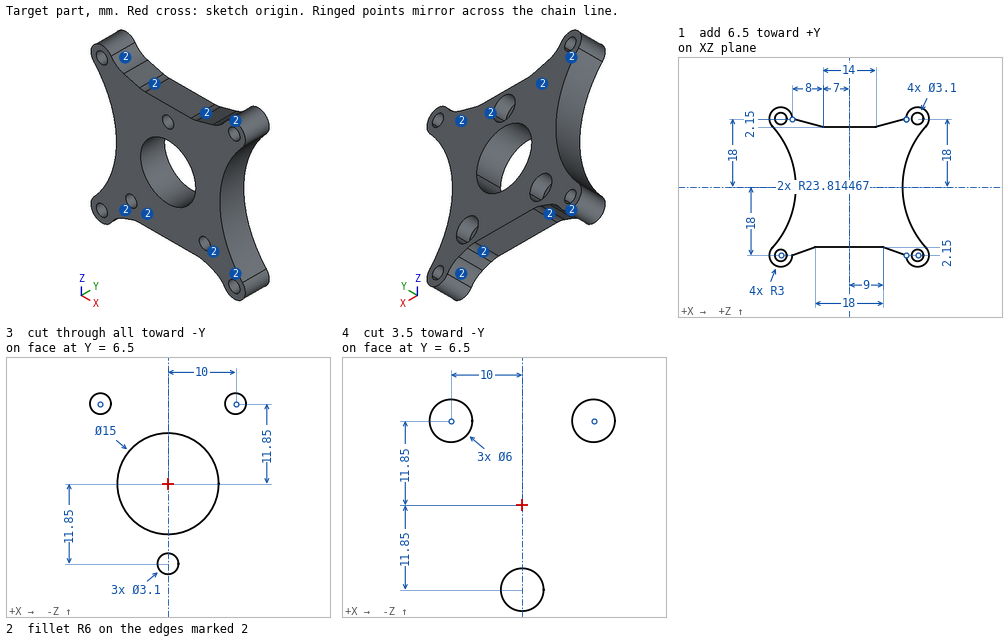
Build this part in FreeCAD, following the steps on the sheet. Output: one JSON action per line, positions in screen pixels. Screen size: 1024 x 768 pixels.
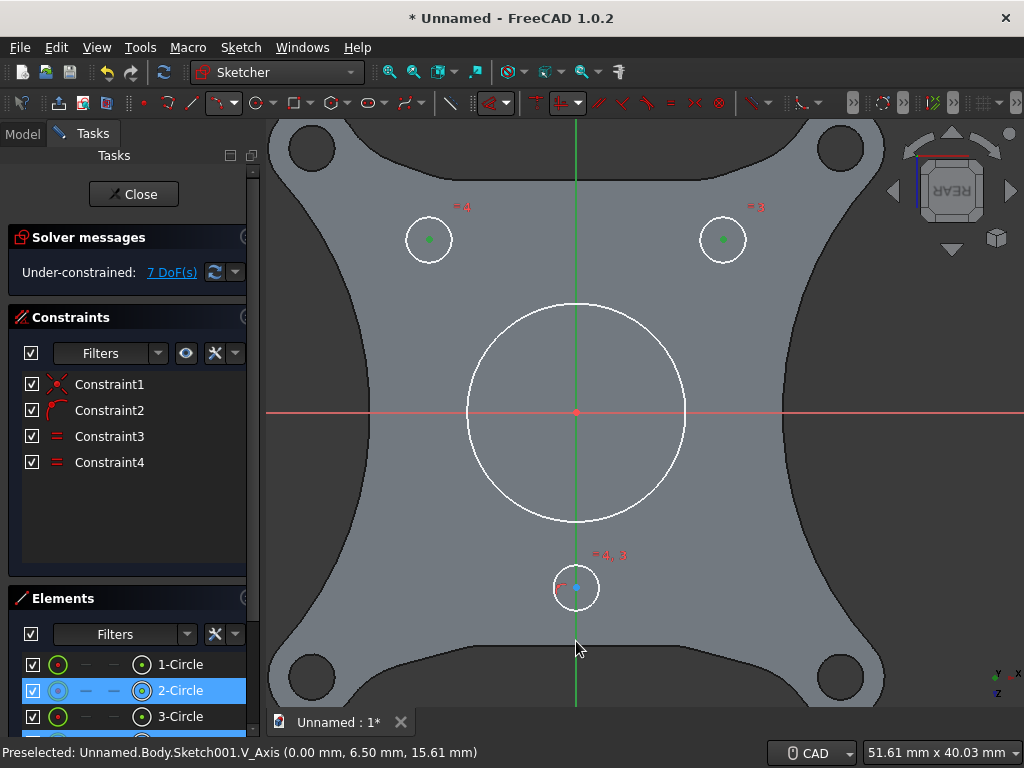
{"action": "left_click", "coordinate": [696, 104]}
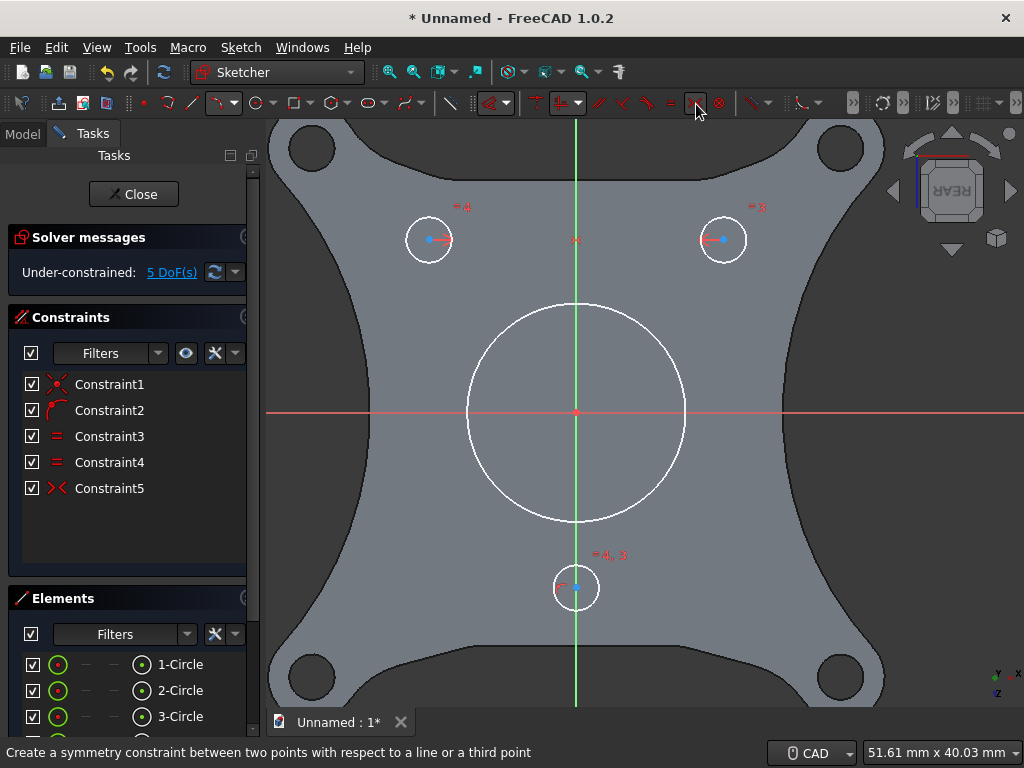
{"action": "left_click", "coordinate": [653, 335]}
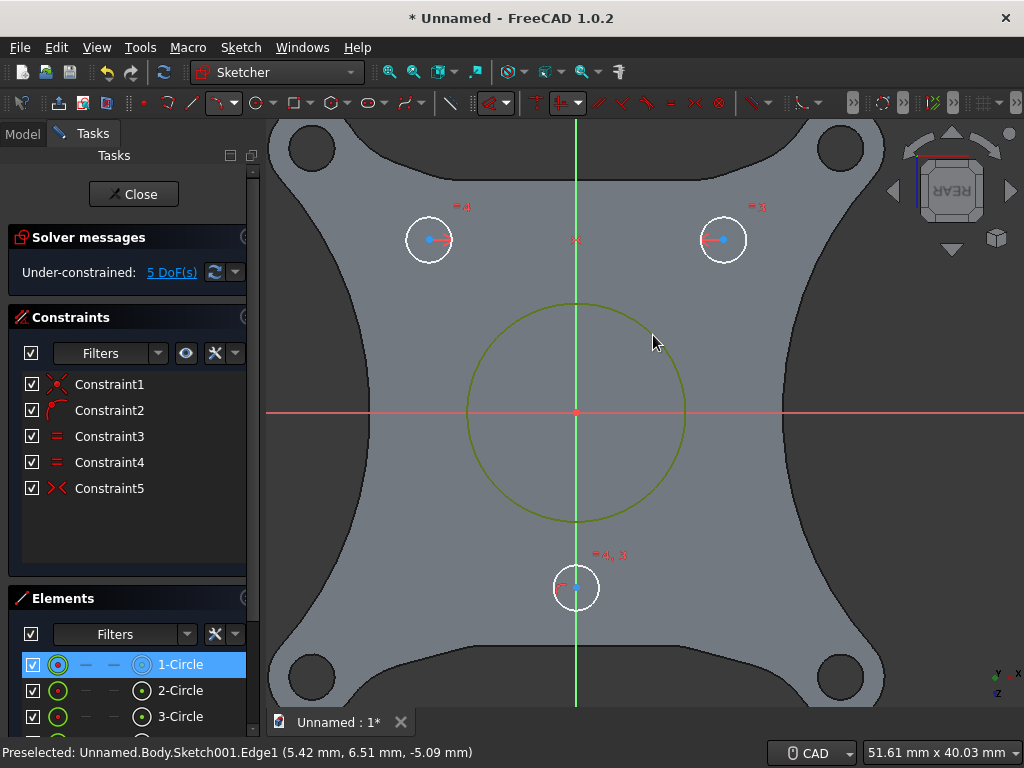
{"action": "key", "text": "k o"}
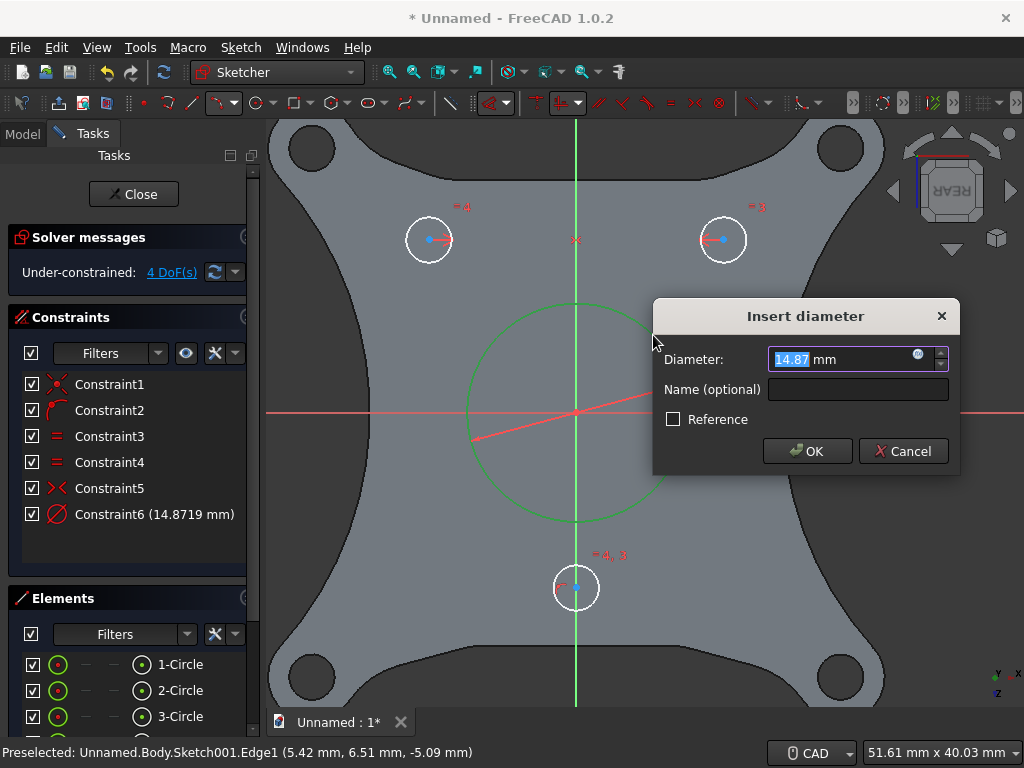
{"action": "type", "text": "15"}
{"action": "key", "text": "Return"}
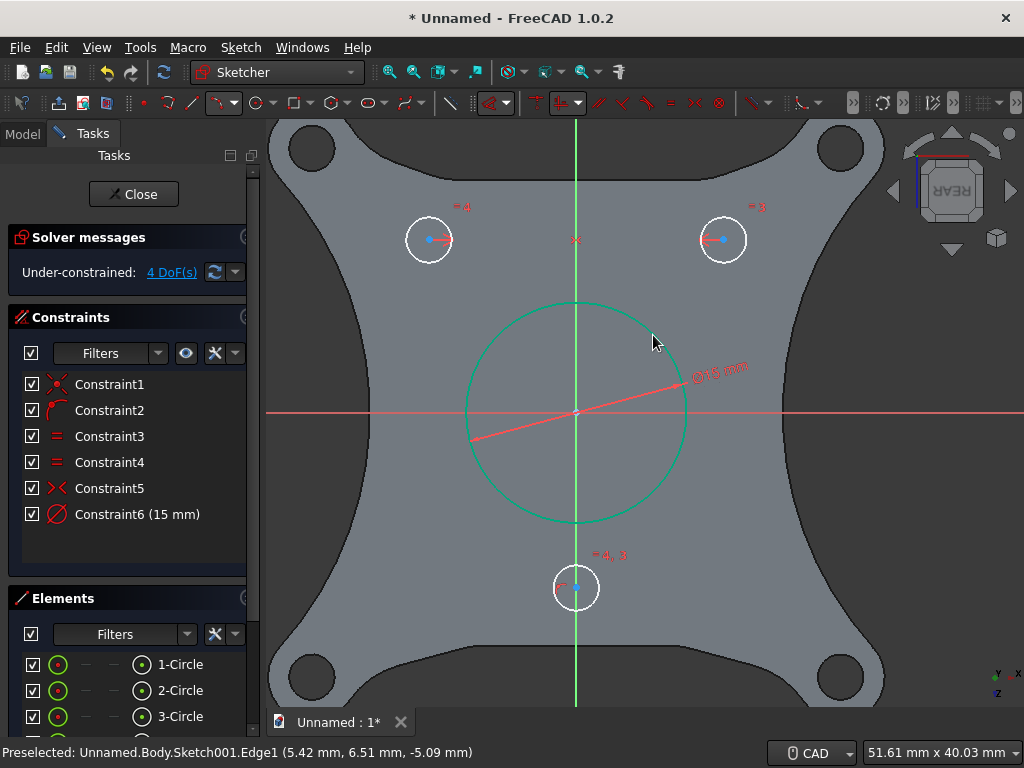
{"action": "left_click", "coordinate": [740, 224]}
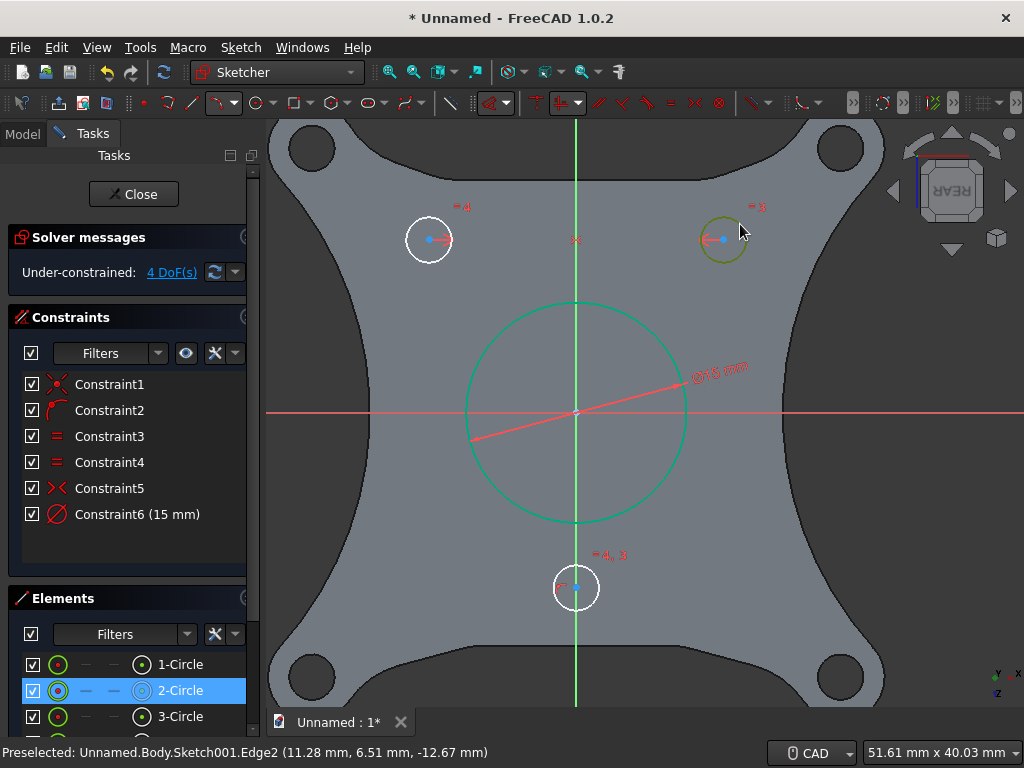
{"action": "left_click", "coordinate": [508, 104]}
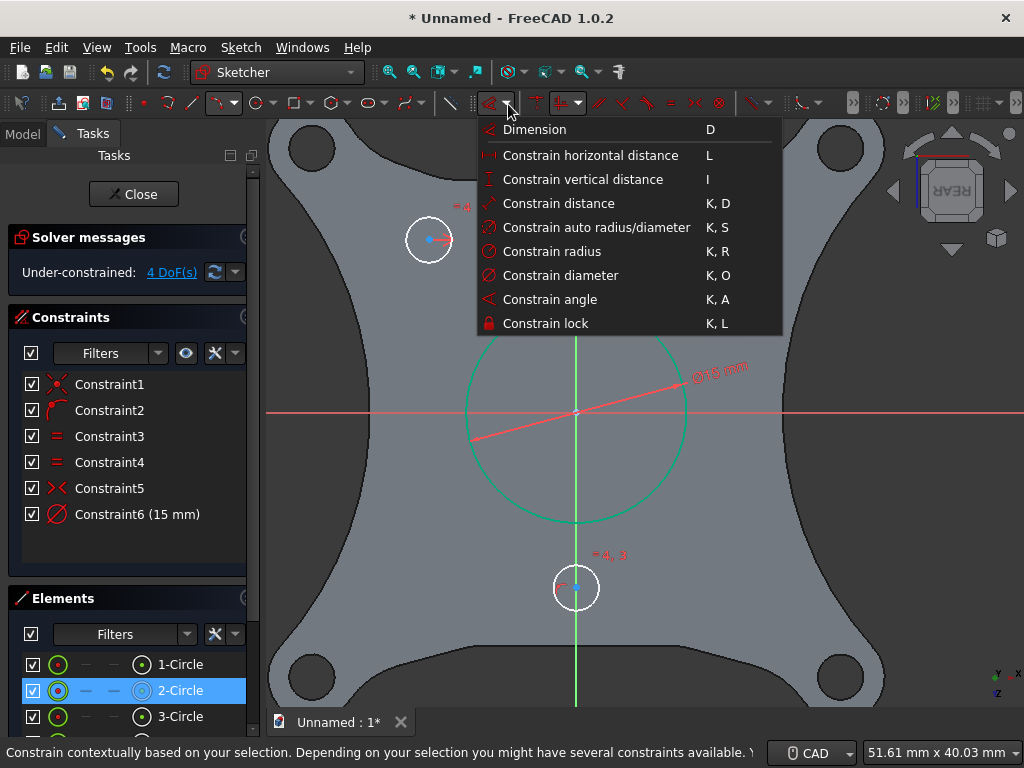
{"action": "left_click", "coordinate": [630, 275]}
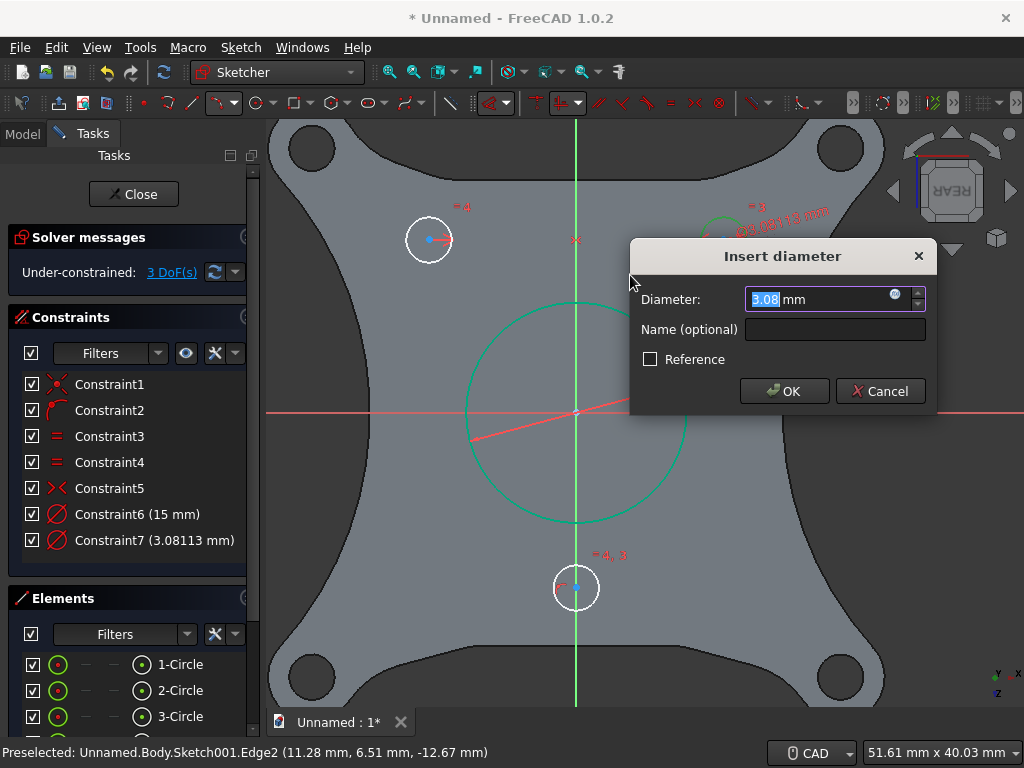
{"action": "type", "text": "3.1"}
{"action": "key", "text": "Return"}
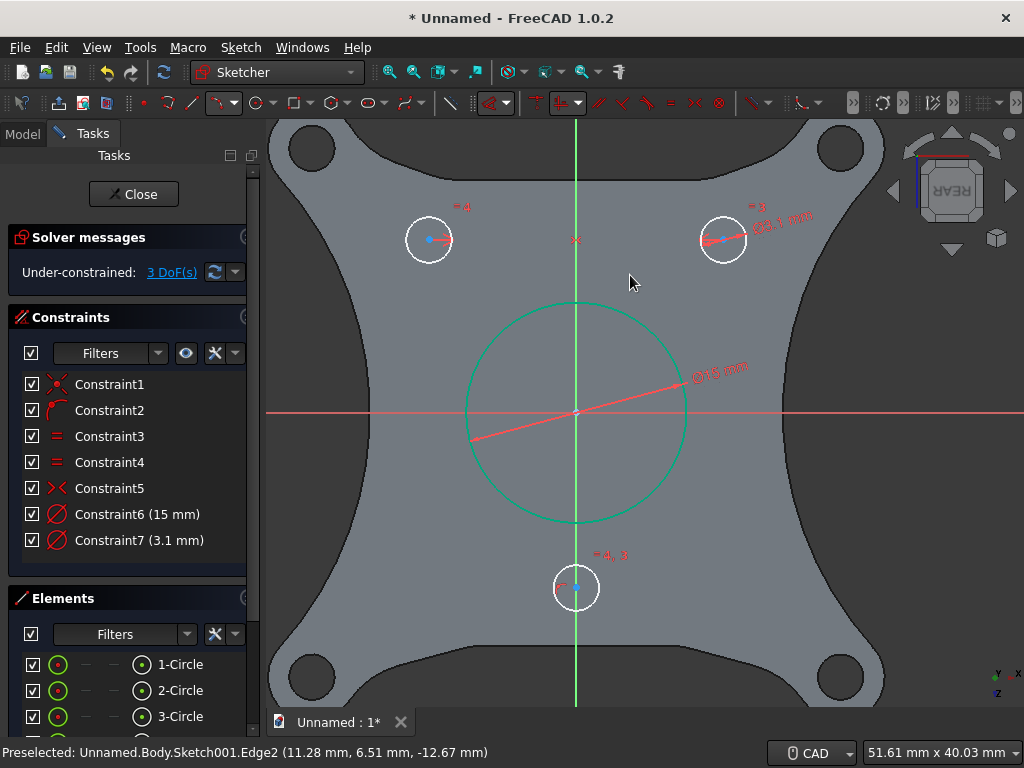
{"action": "left_click", "coordinate": [724, 240]}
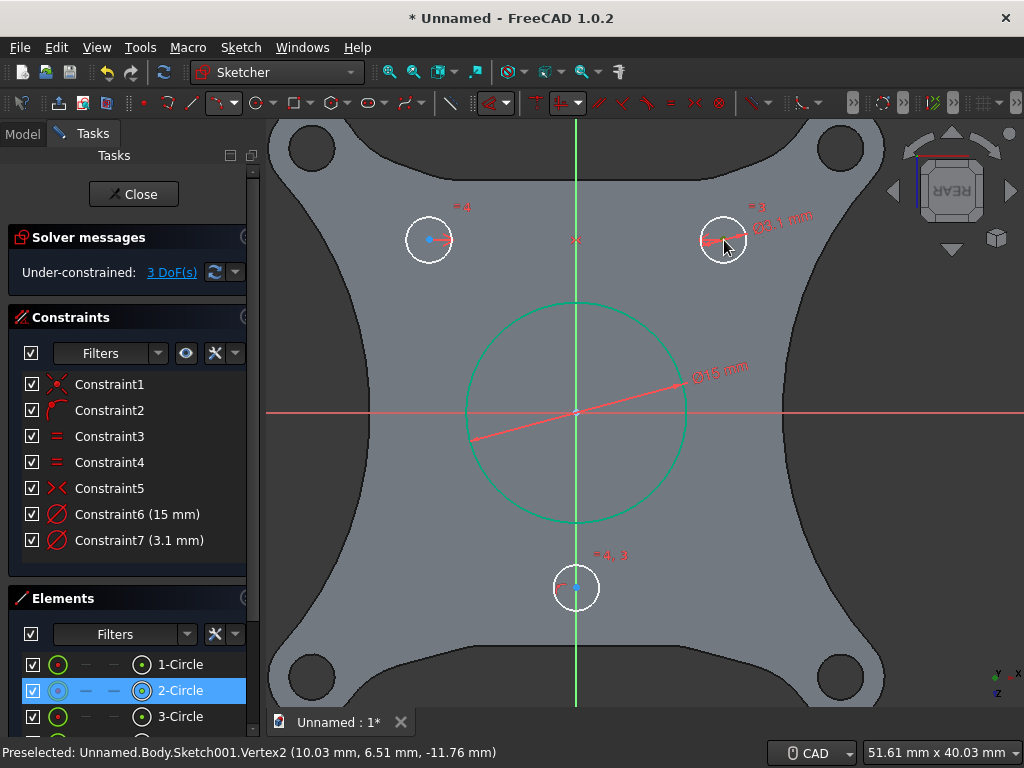
{"action": "left_click", "coordinate": [508, 104]}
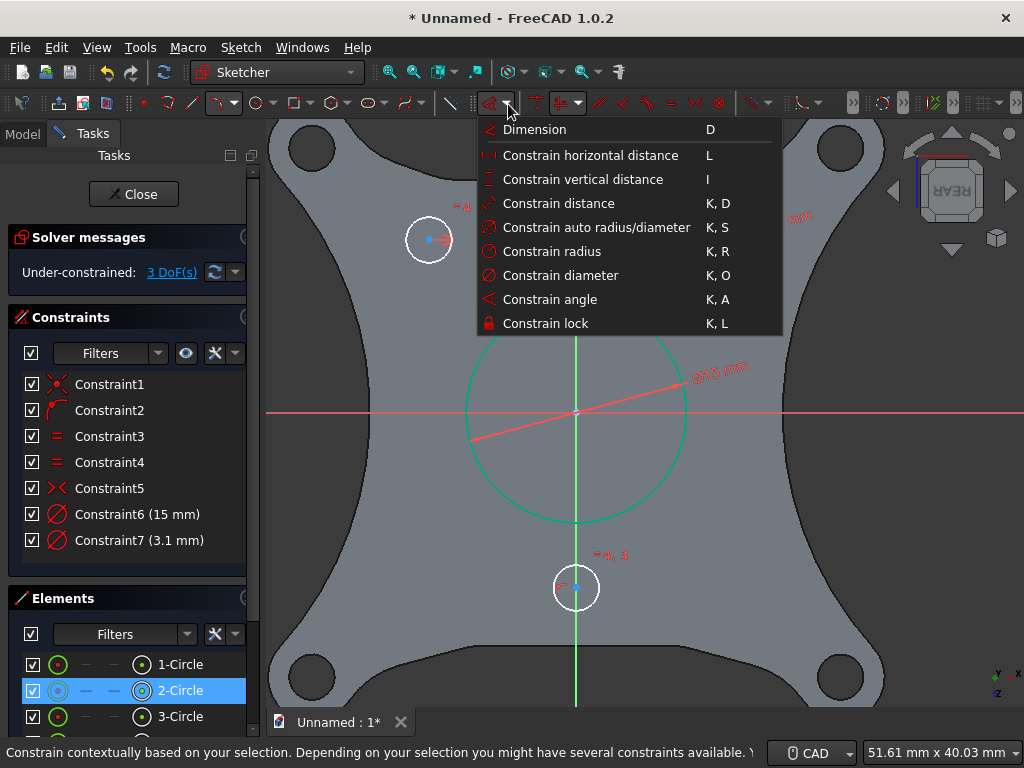
{"action": "left_click", "coordinate": [630, 155]}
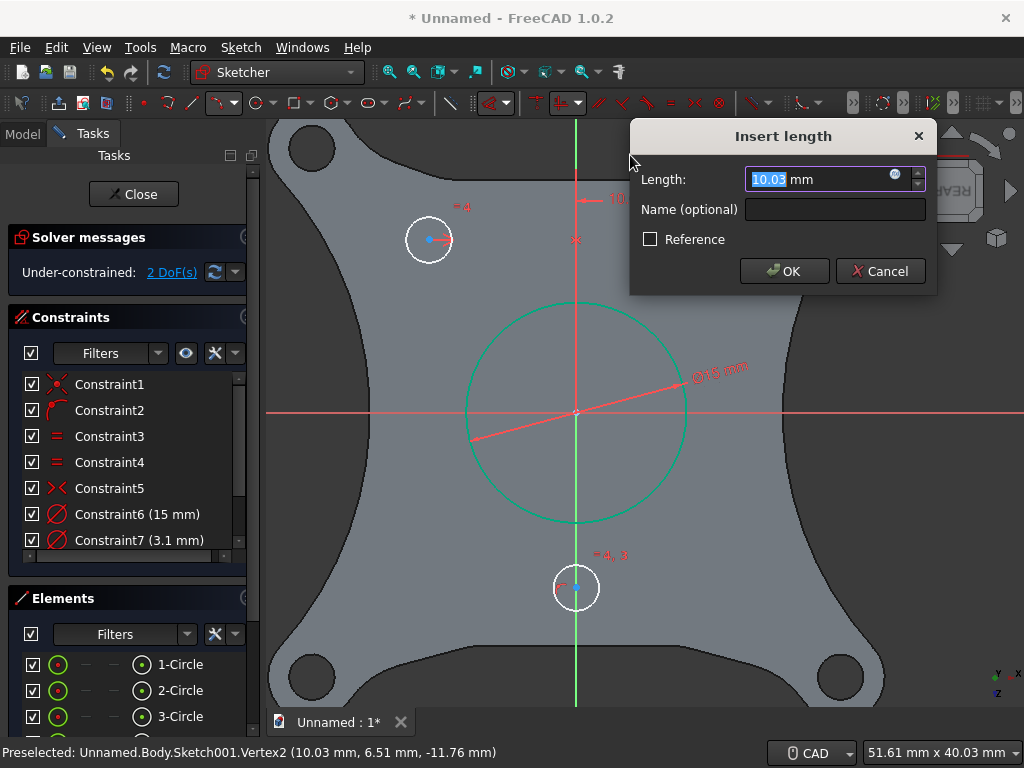
{"action": "type", "text": "10"}
{"action": "key", "text": "Return"}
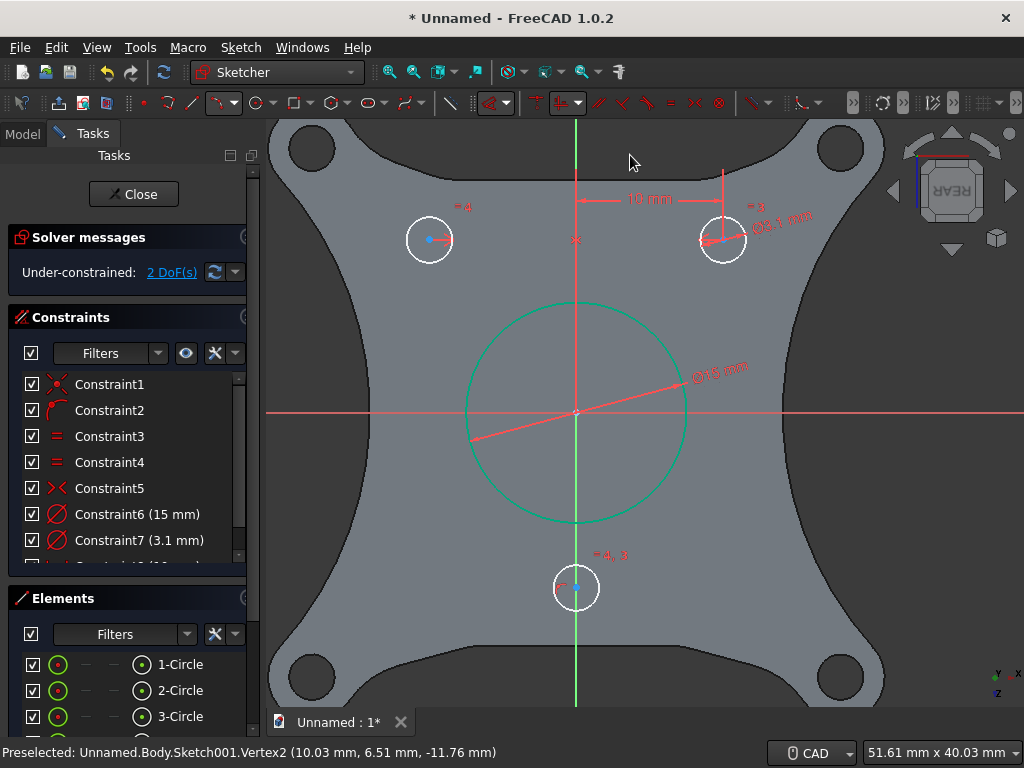
{"action": "left_click", "coordinate": [723, 240]}